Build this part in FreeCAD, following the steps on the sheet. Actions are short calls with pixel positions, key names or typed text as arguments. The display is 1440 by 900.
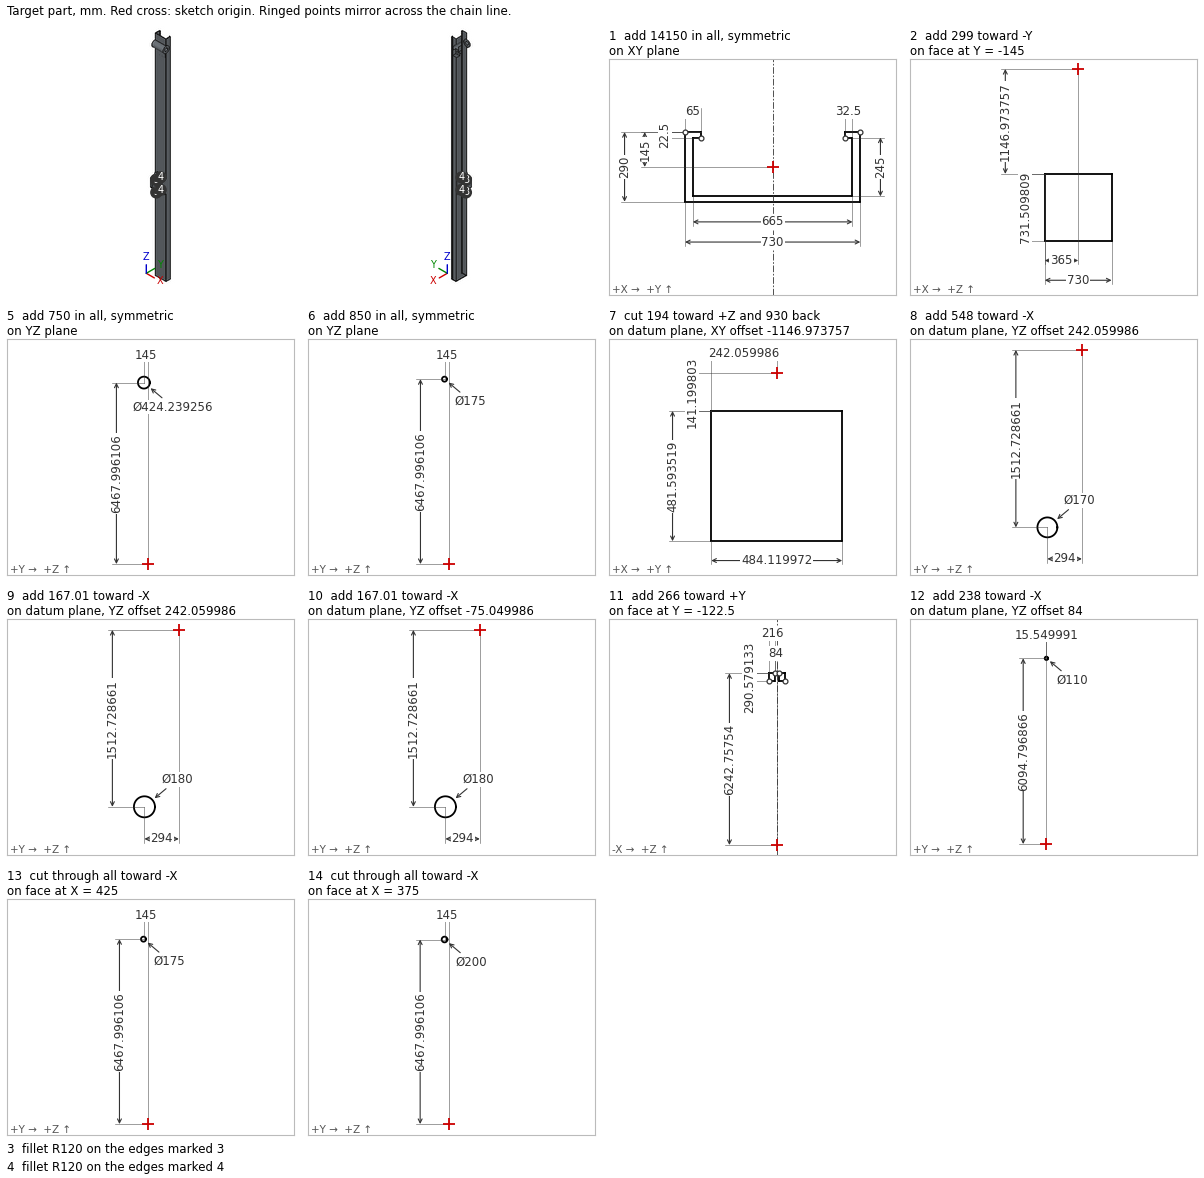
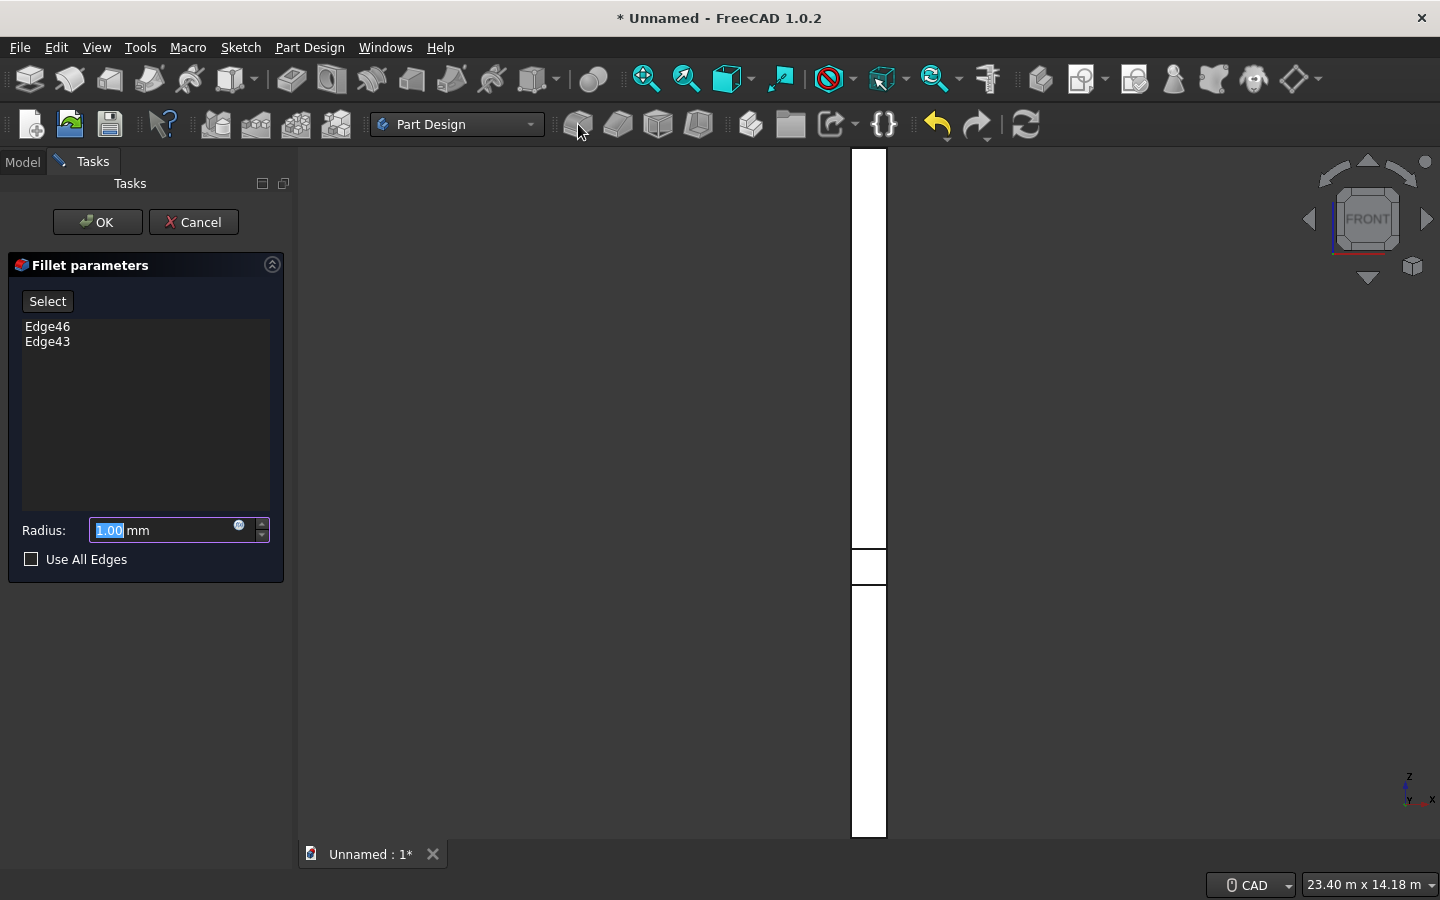
text(120)
key(Tab)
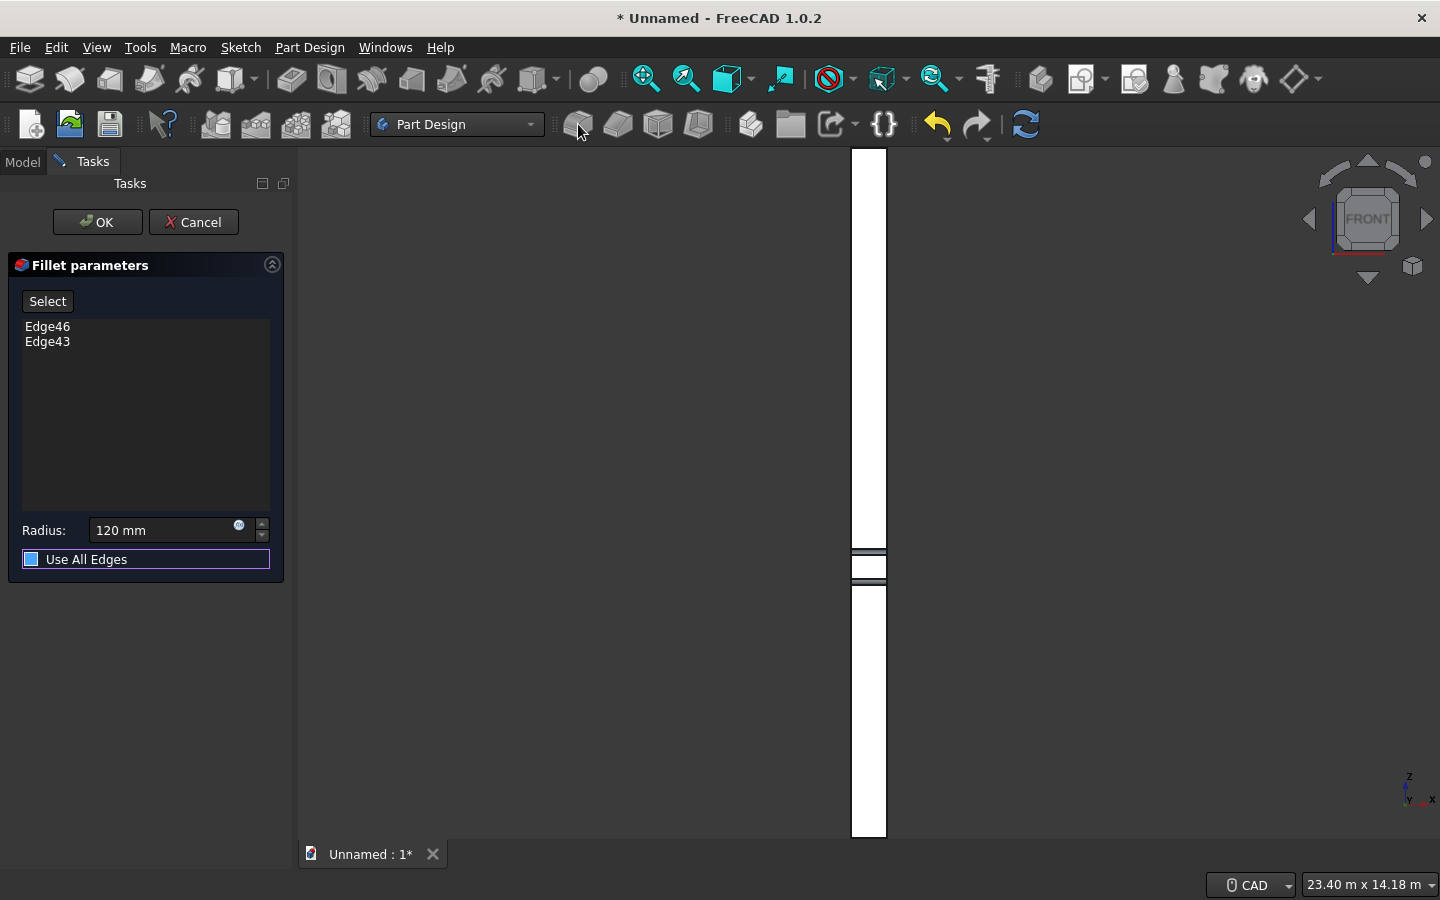
click(98, 222)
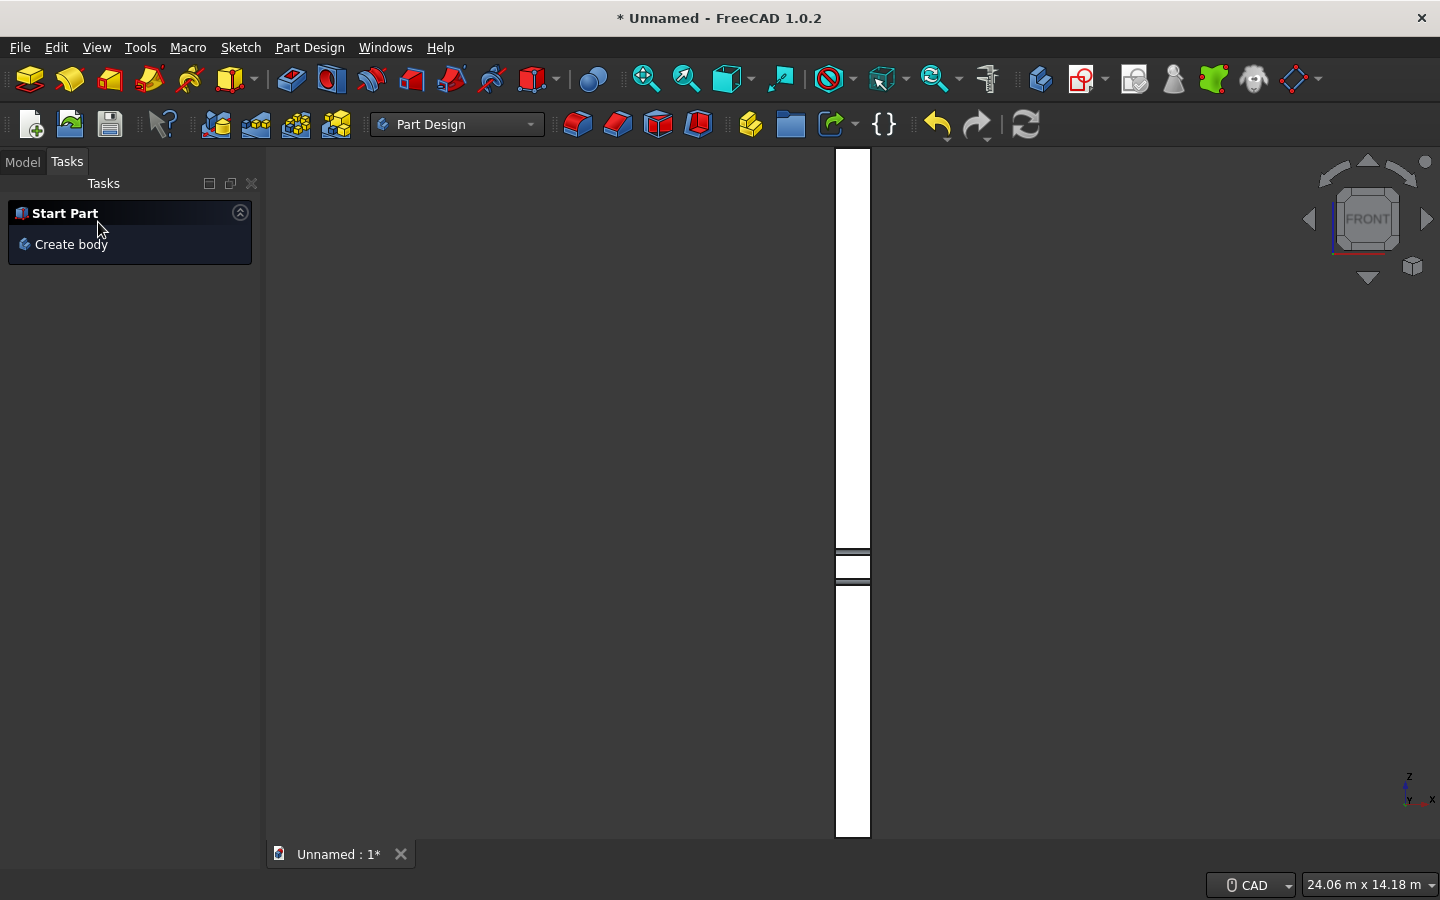
key(0)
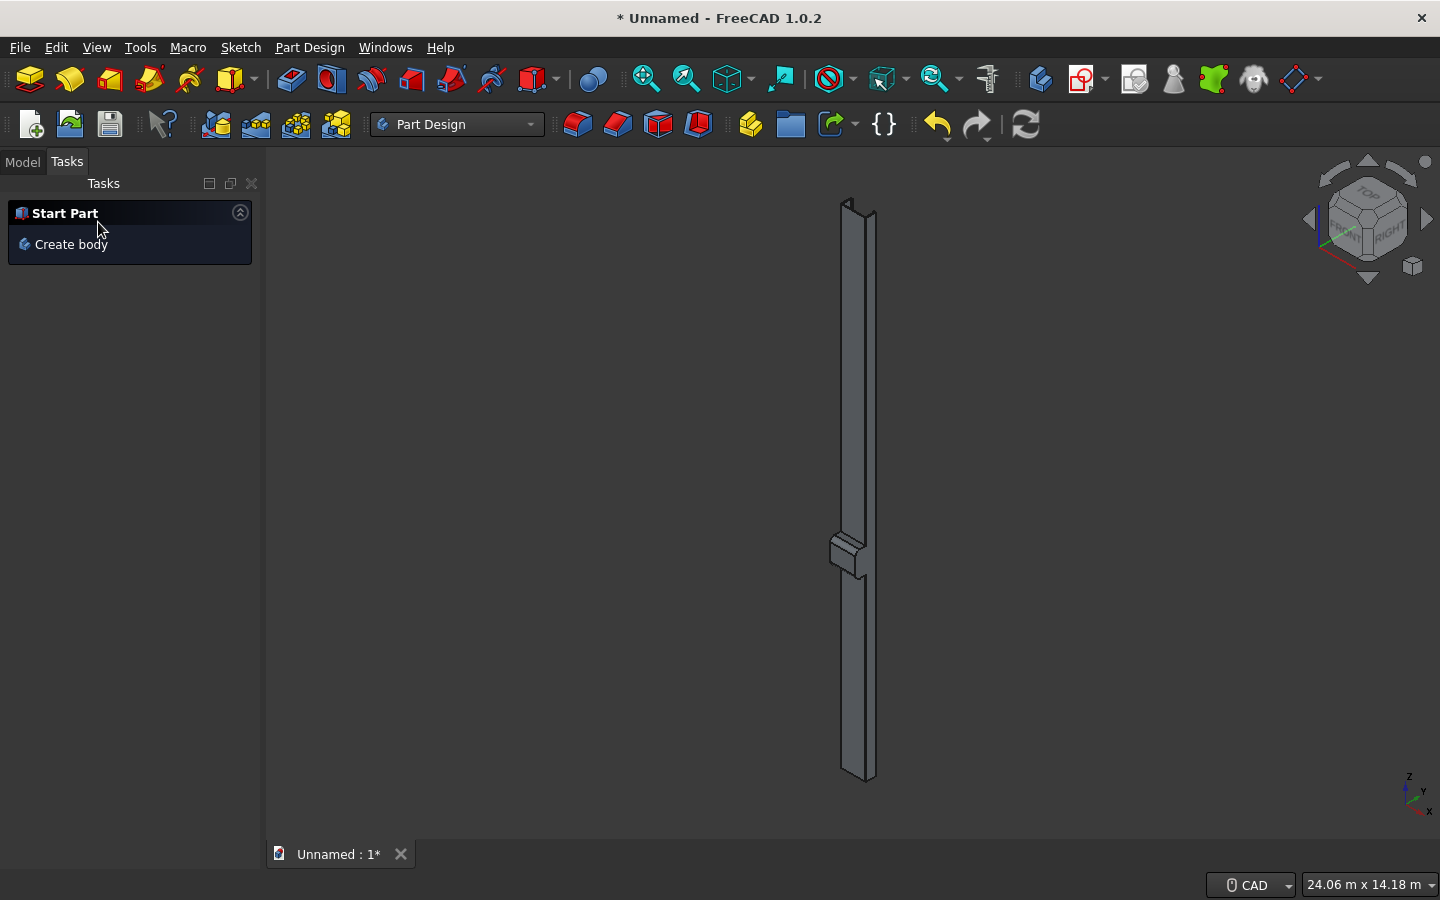
key(2)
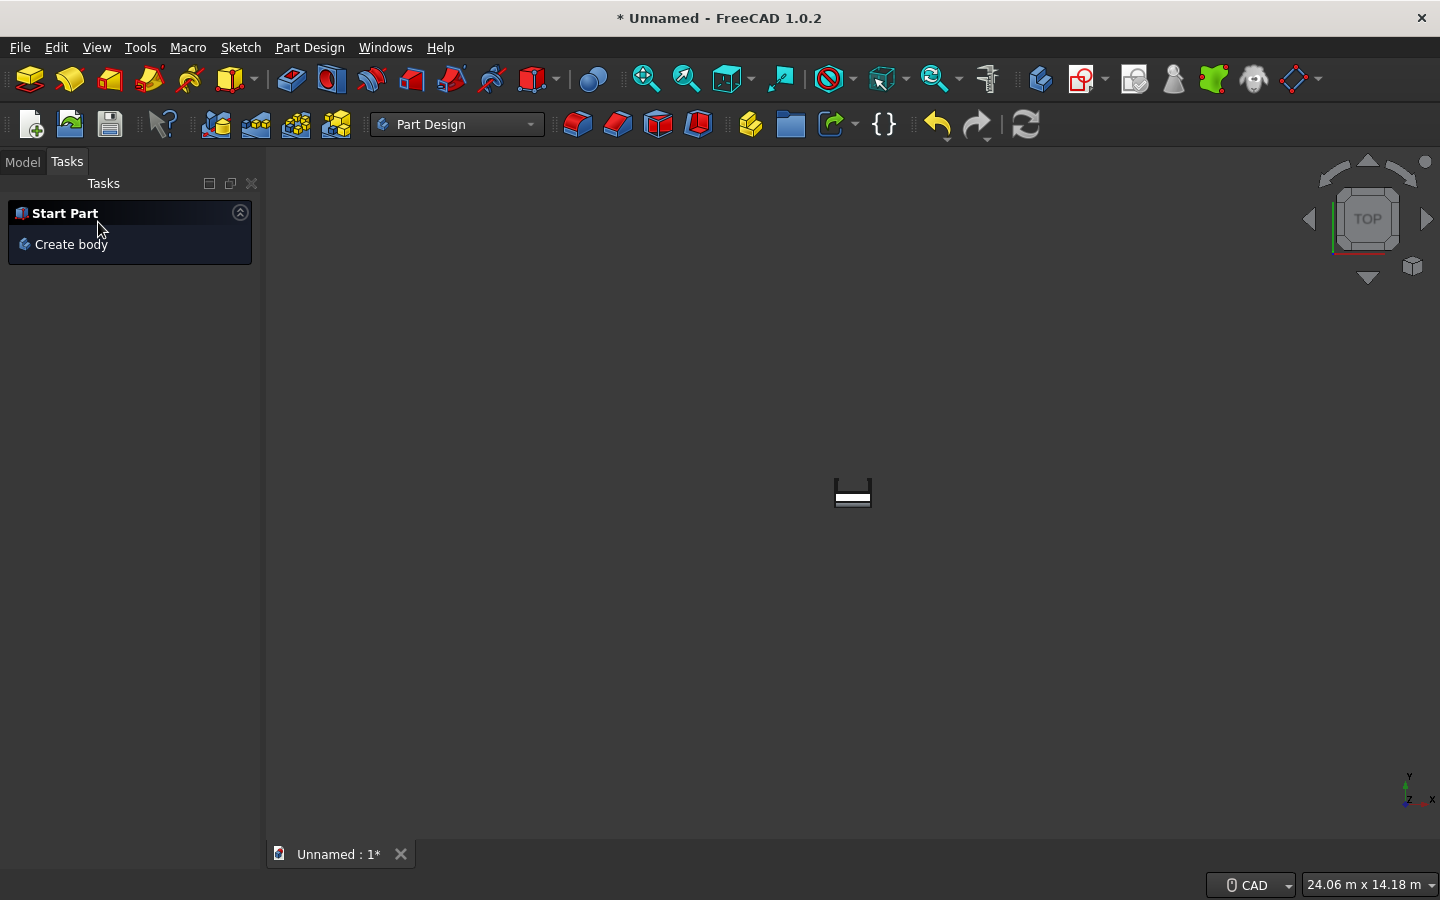
key(v)
key(f)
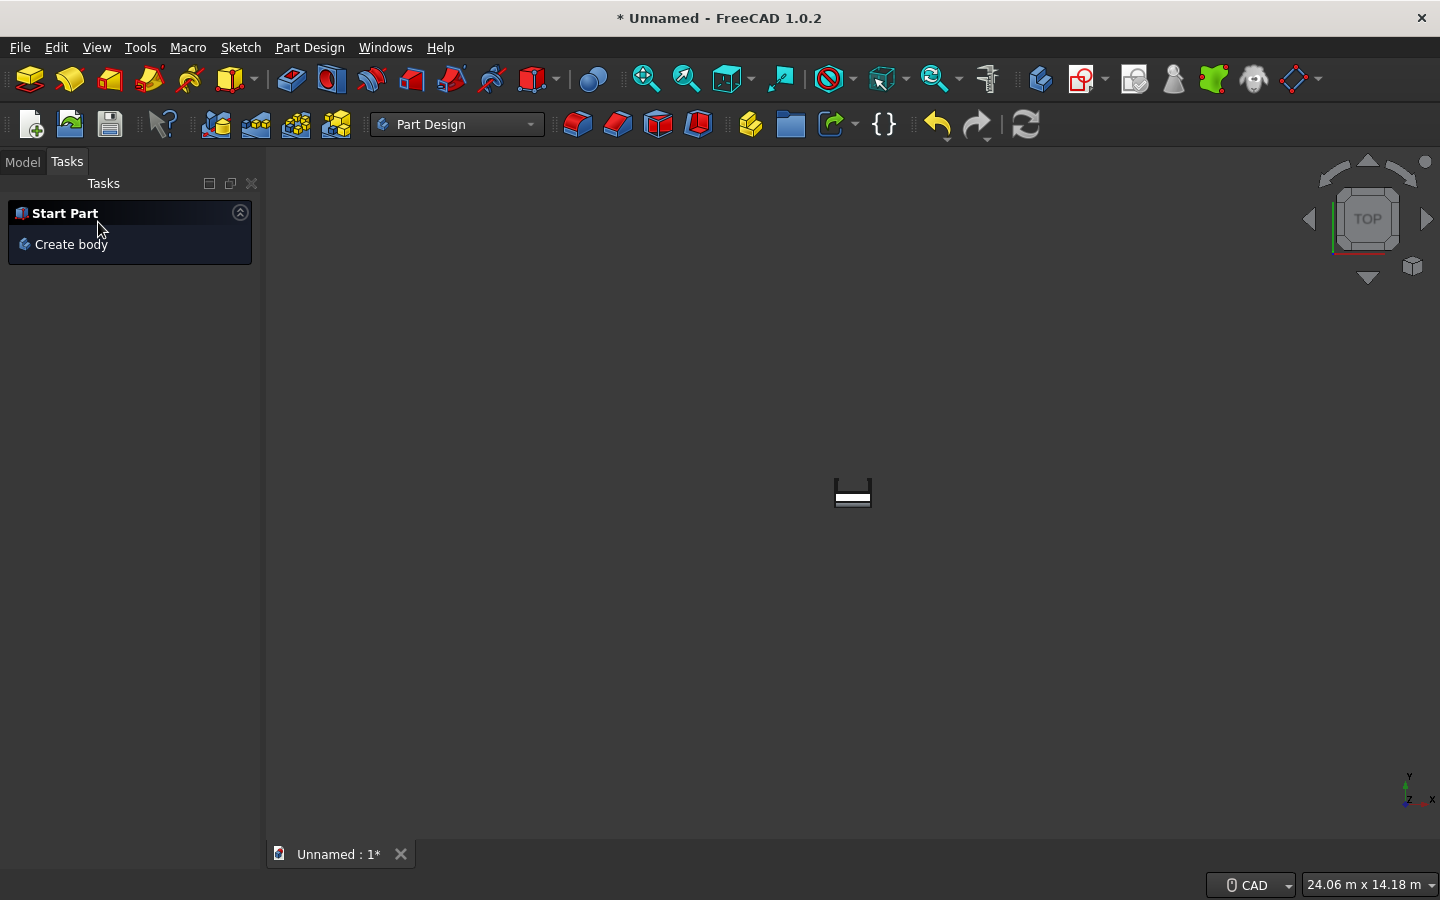
key(1)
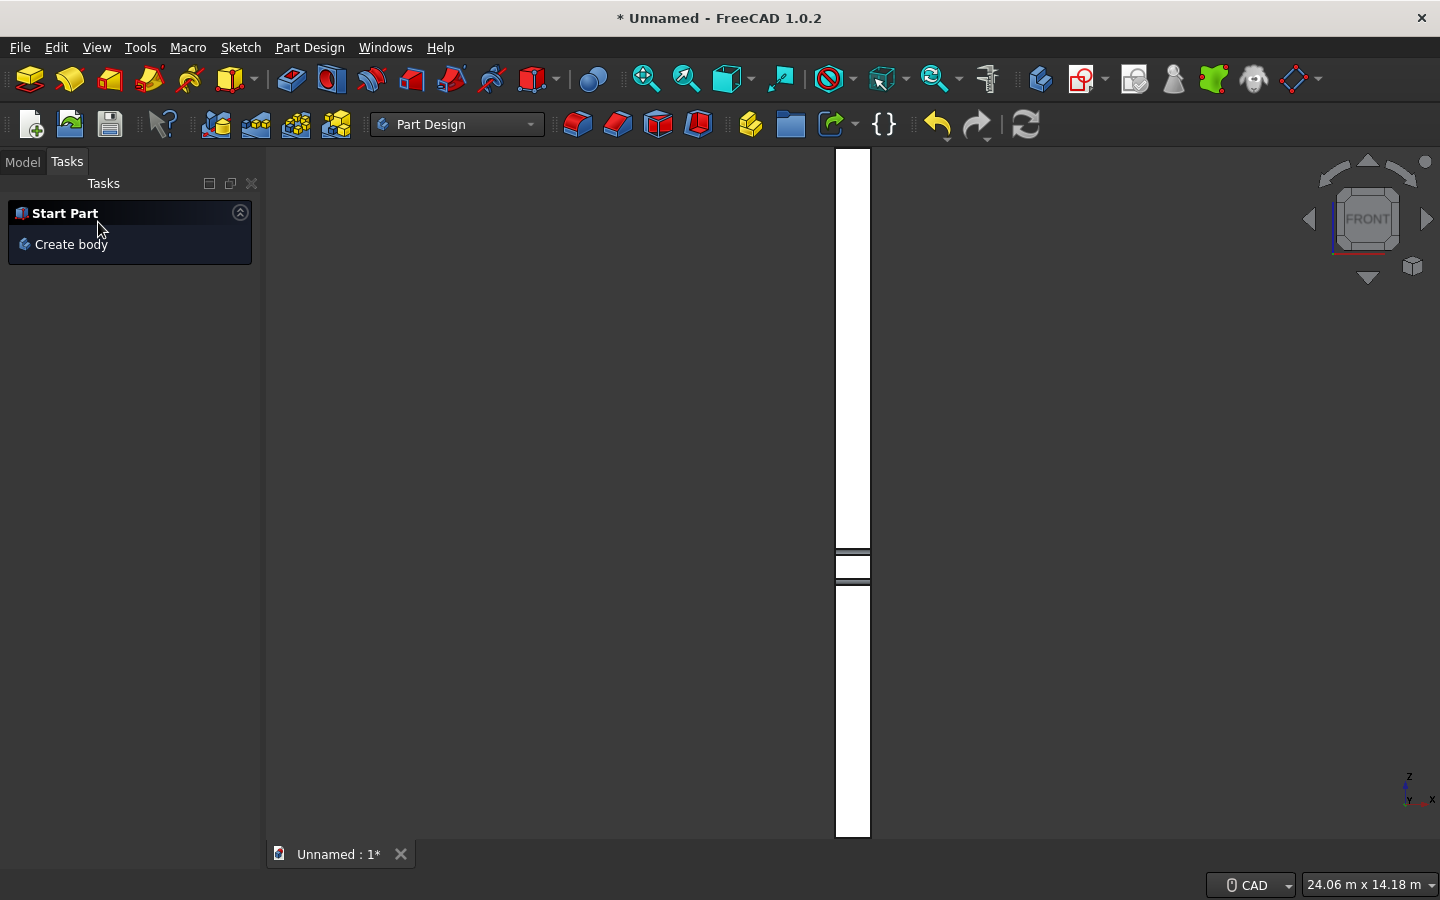
key(3)